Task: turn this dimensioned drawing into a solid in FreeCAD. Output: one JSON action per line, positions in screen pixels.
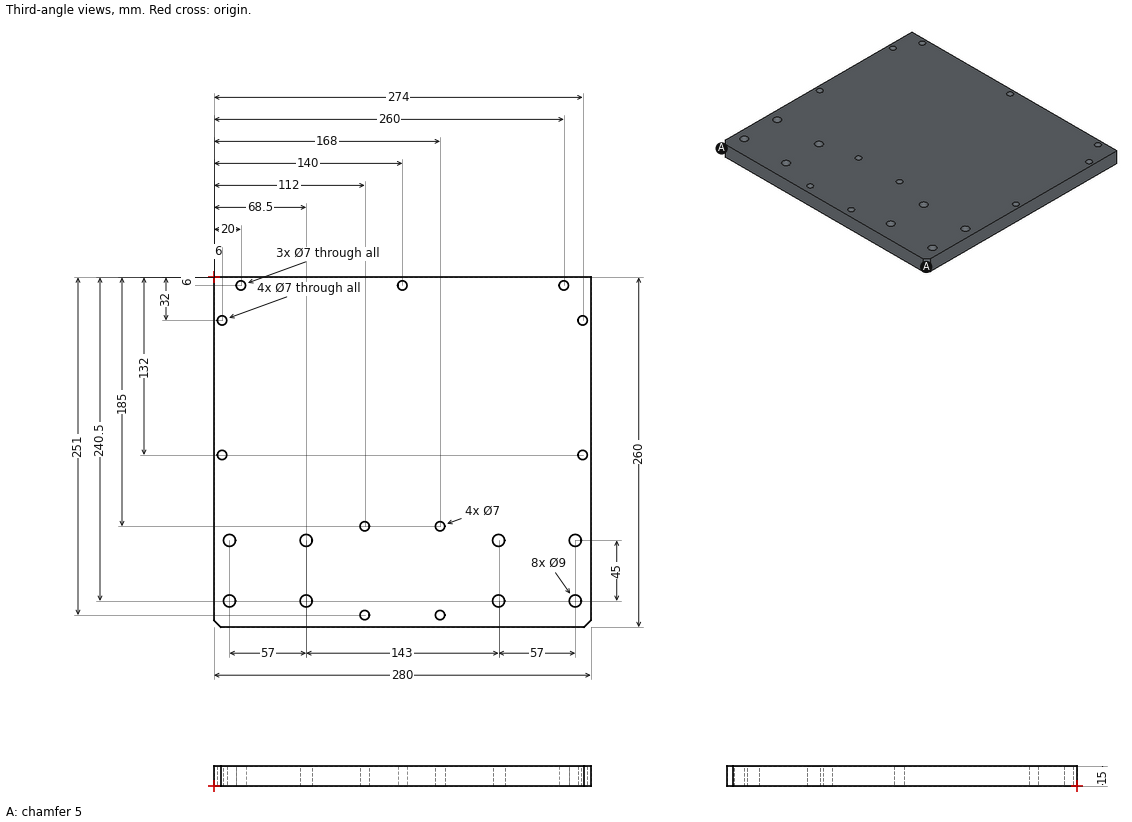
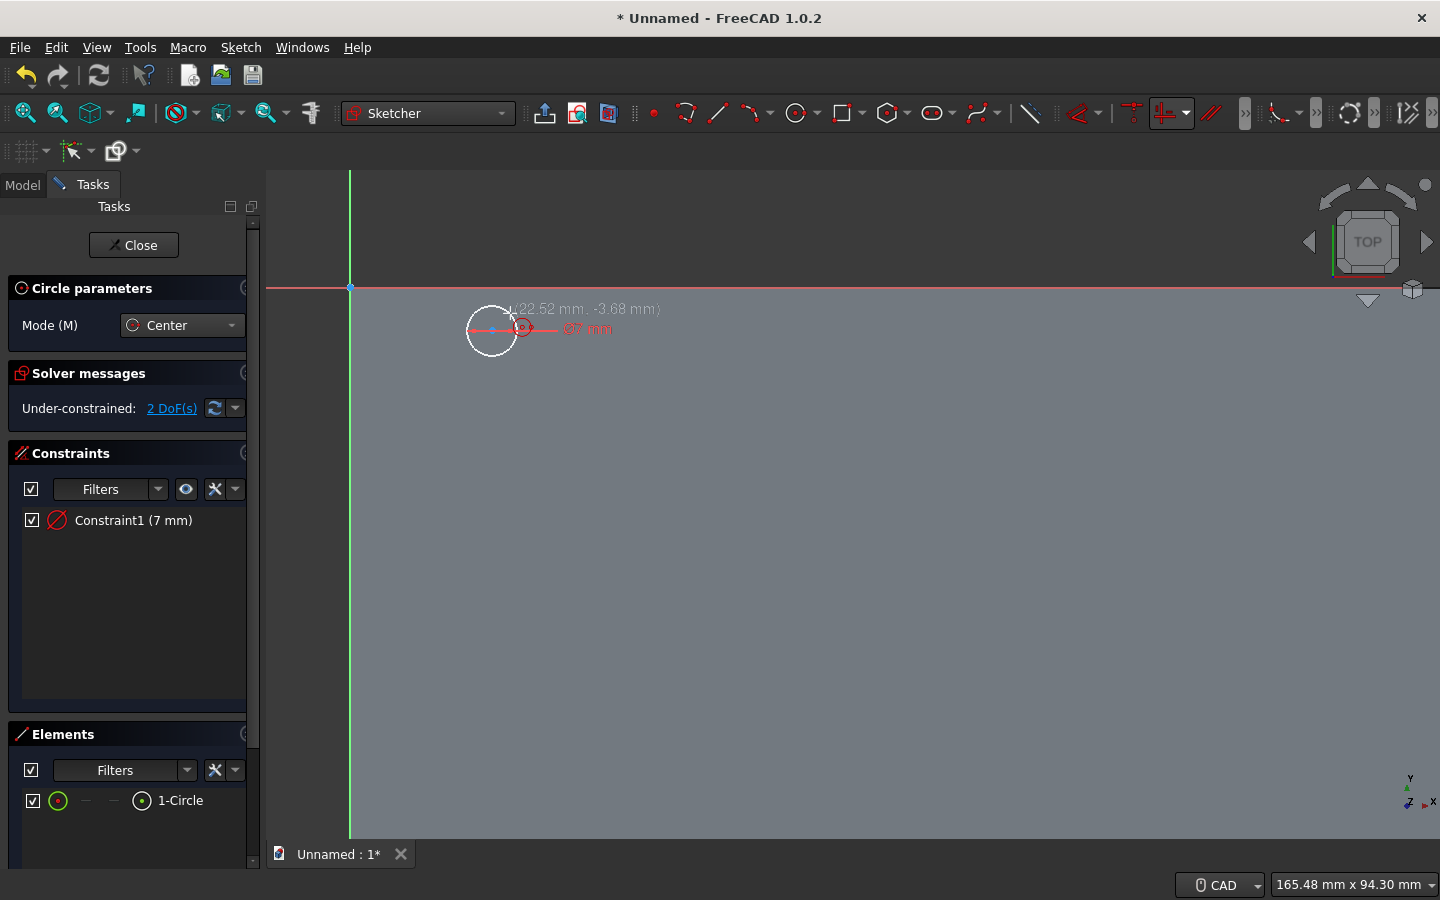
{"action": "scroll", "coordinate": [493, 611], "scroll_direction": "down", "scroll_amount": 5}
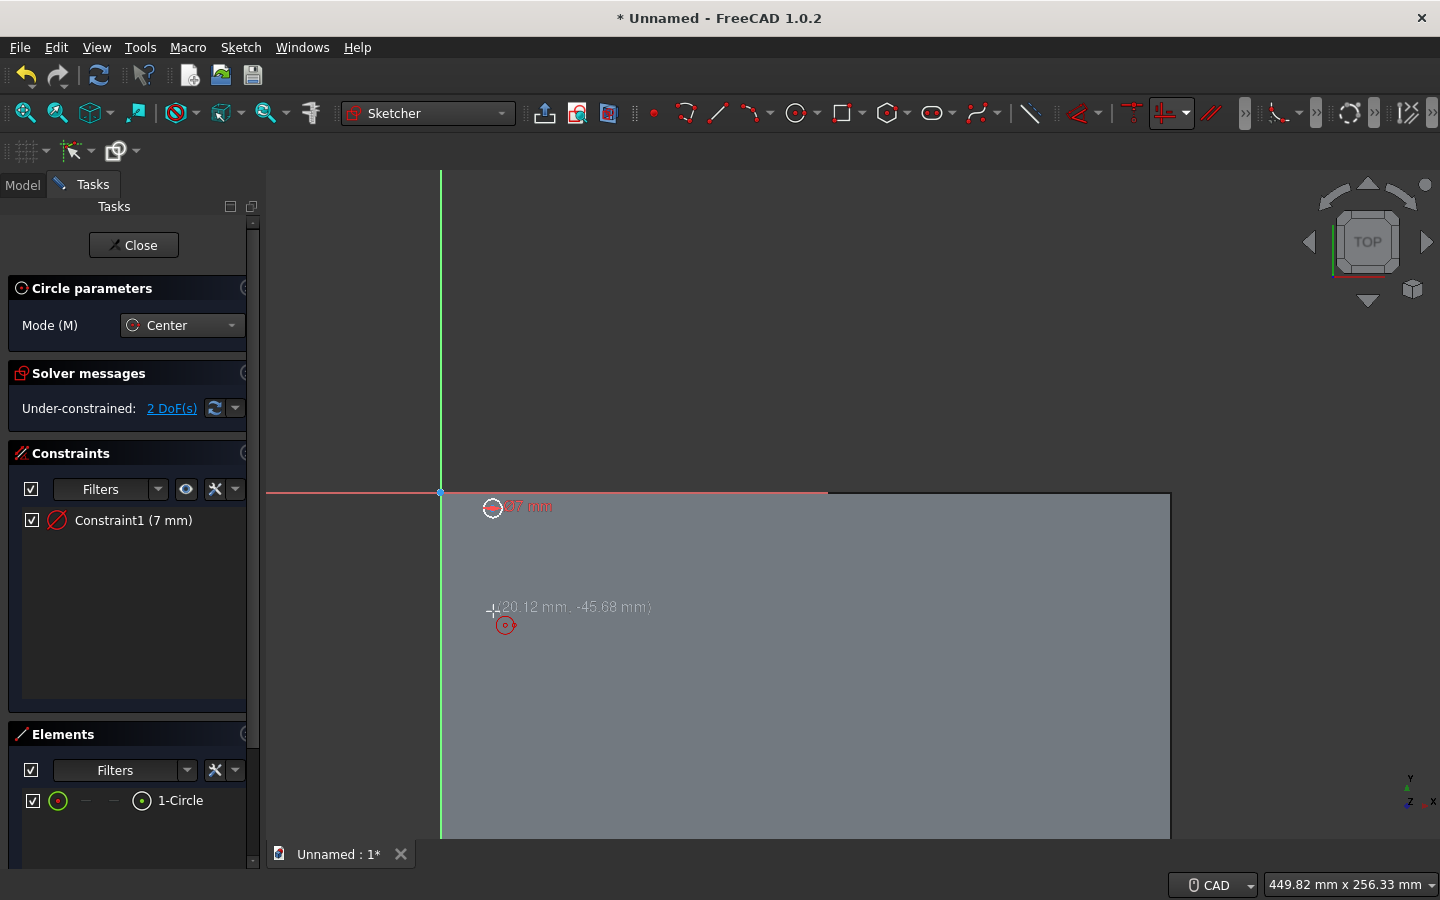
{"action": "scroll", "coordinate": [1119, 508], "scroll_direction": "up", "scroll_amount": 5}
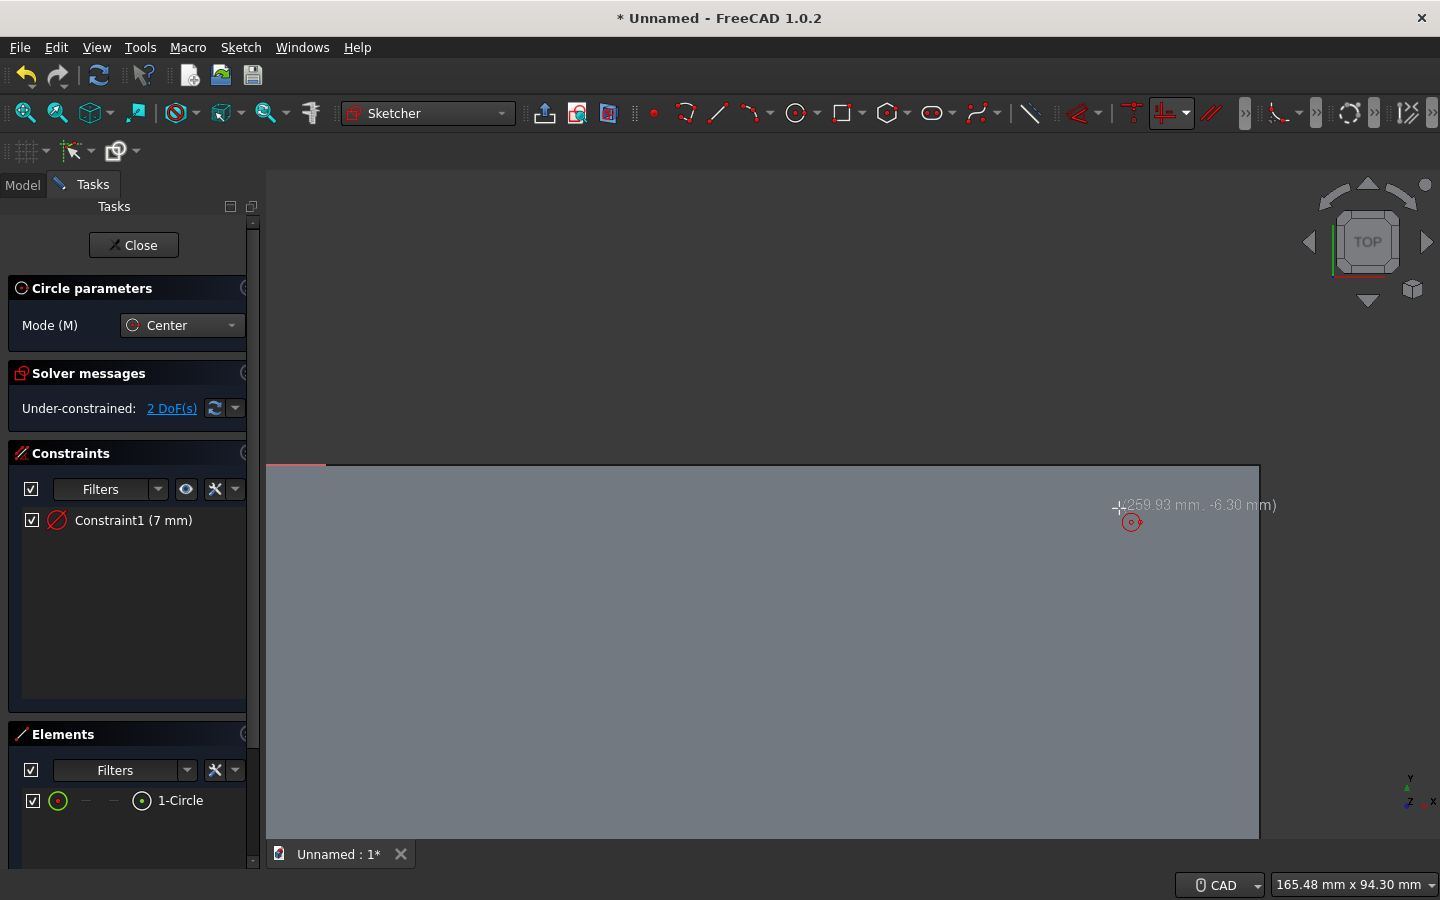
{"action": "left_click", "coordinate": [1118, 508]}
{"action": "mouse_move", "coordinate": [1136, 490]}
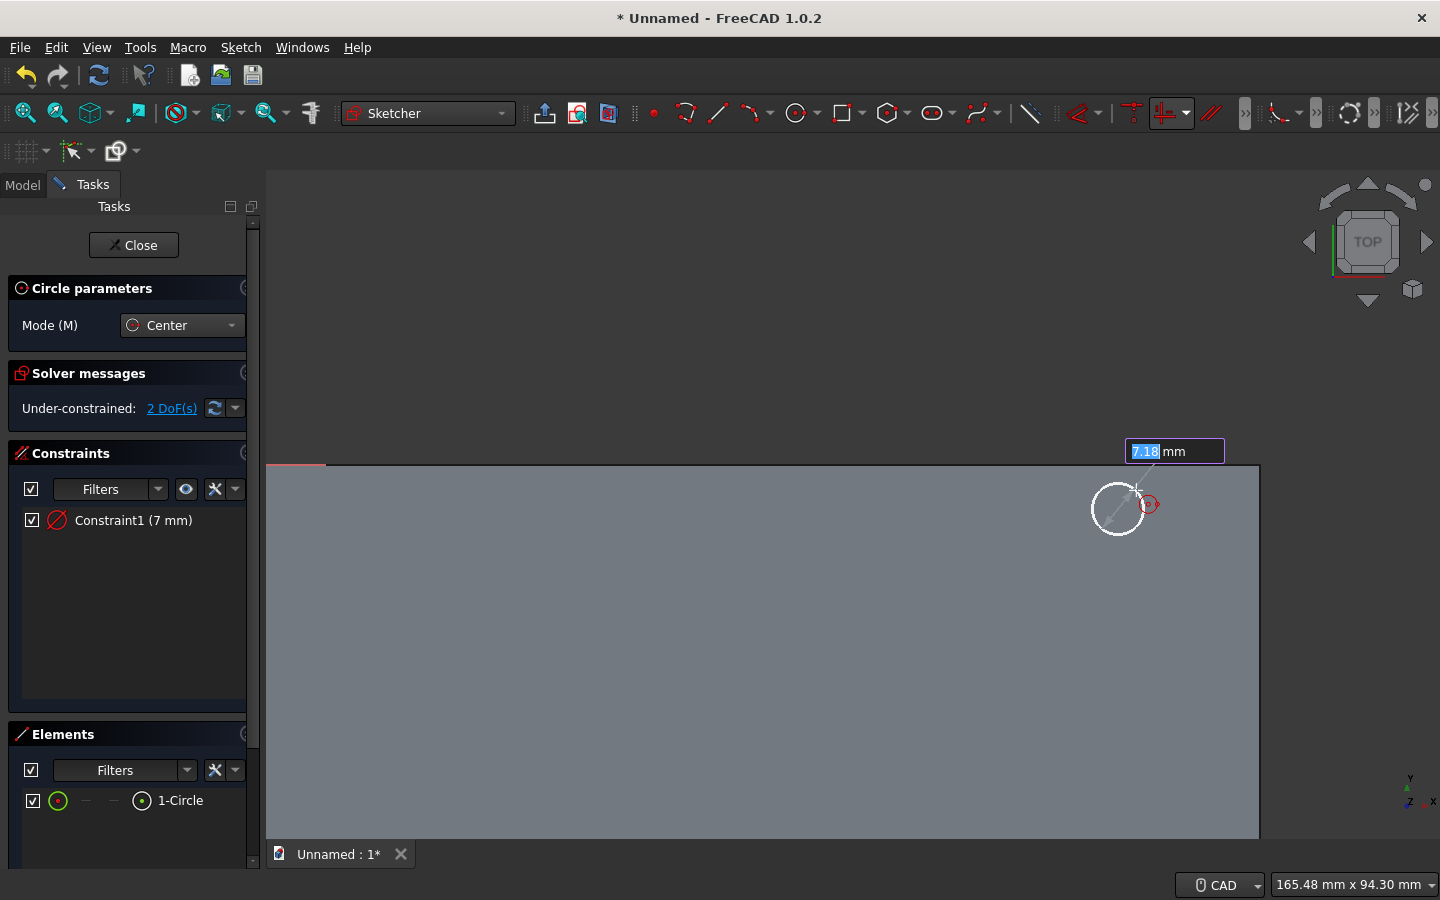
{"action": "type", "text": "7"}
{"action": "key", "text": "Return"}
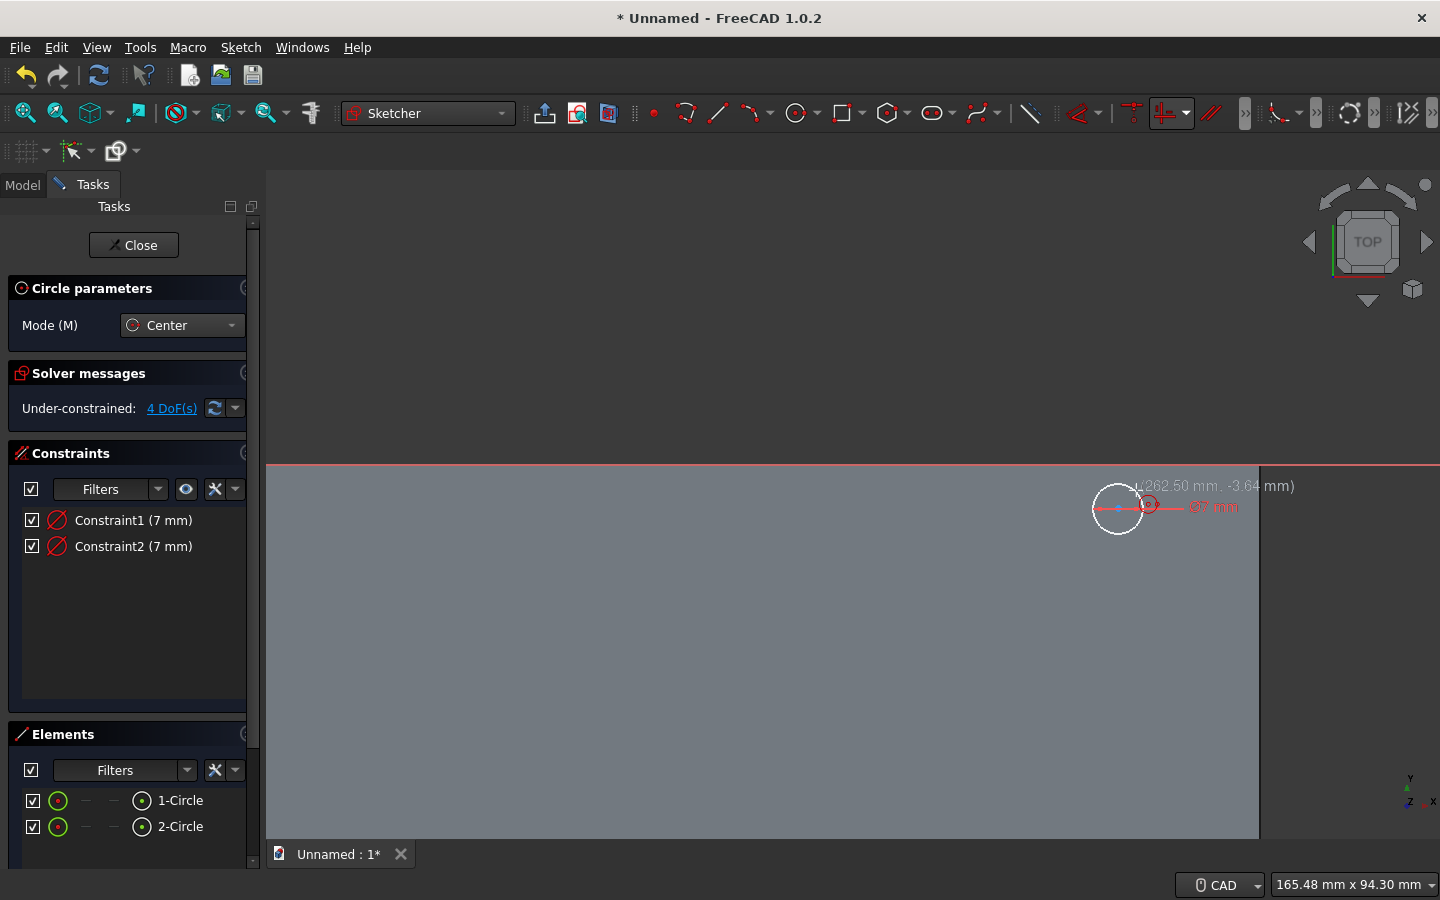
{"action": "scroll", "coordinate": [1120, 508], "scroll_direction": "down", "scroll_amount": 5}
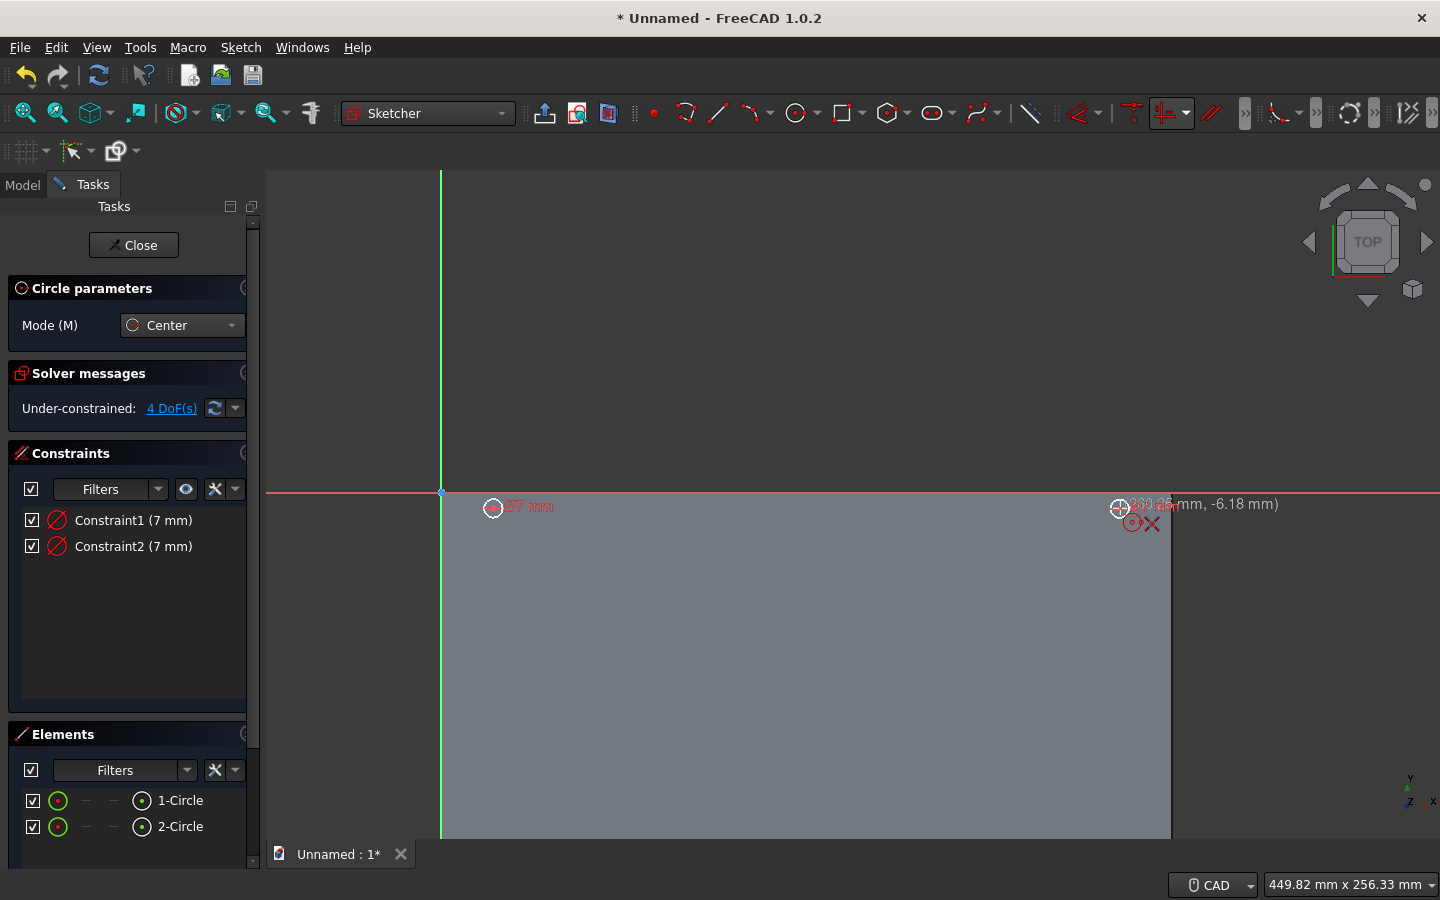
{"action": "scroll", "coordinate": [807, 508], "scroll_direction": "up", "scroll_amount": 5}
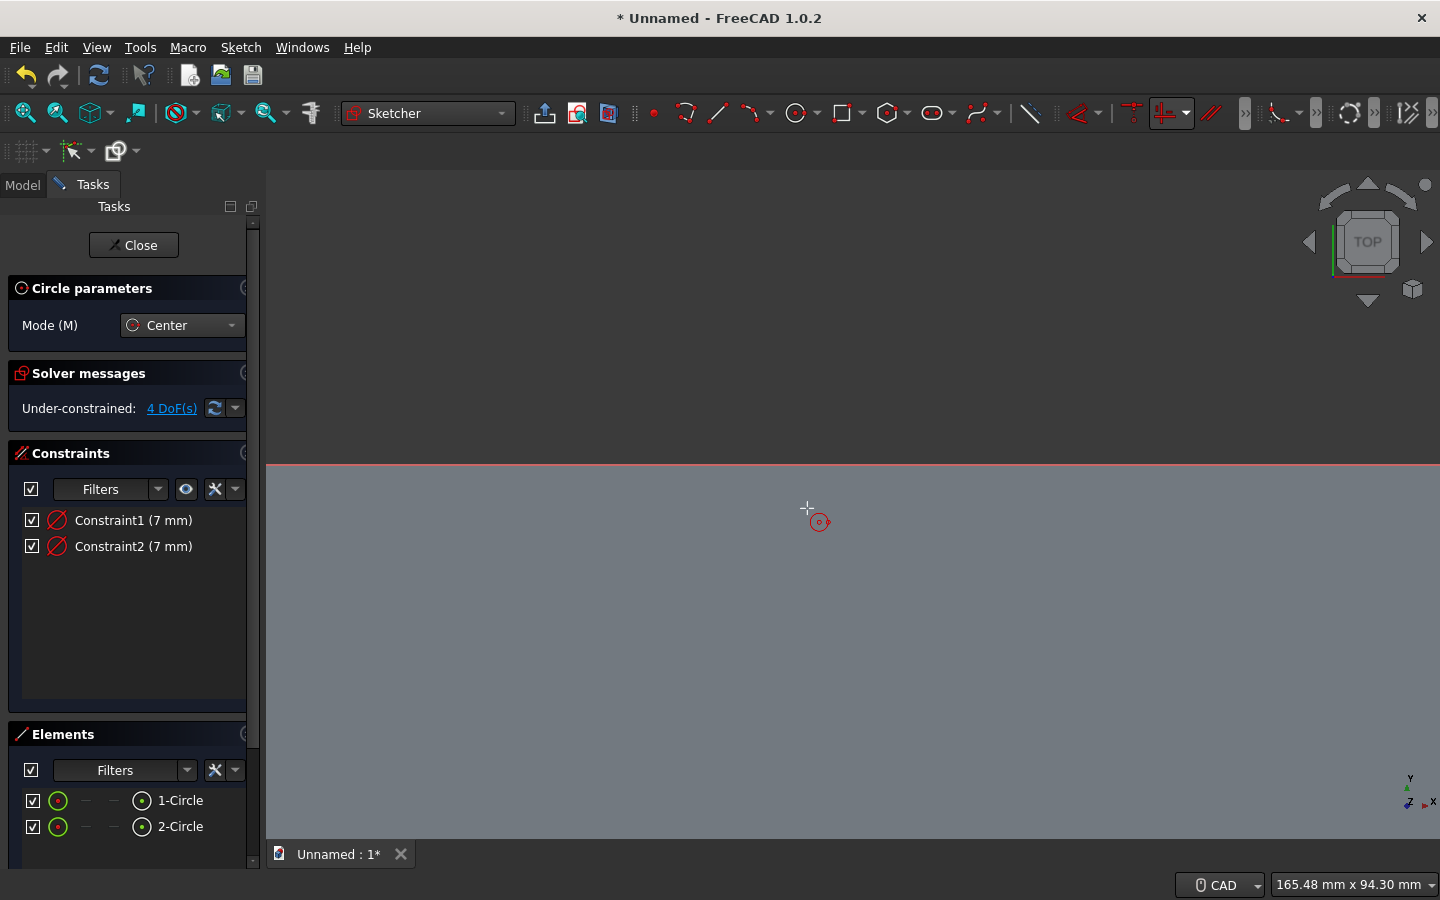
{"action": "left_click", "coordinate": [805, 508]}
{"action": "mouse_move", "coordinate": [823, 490]}